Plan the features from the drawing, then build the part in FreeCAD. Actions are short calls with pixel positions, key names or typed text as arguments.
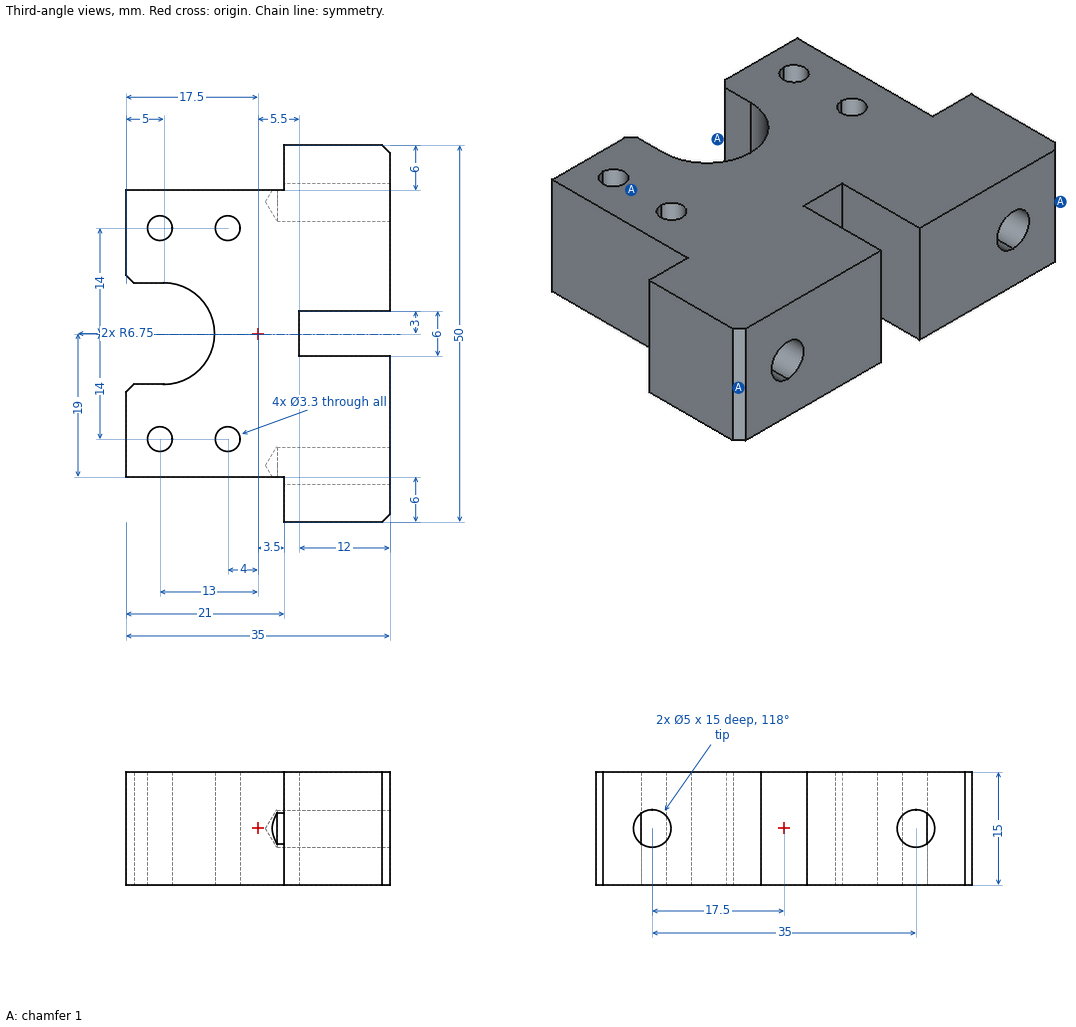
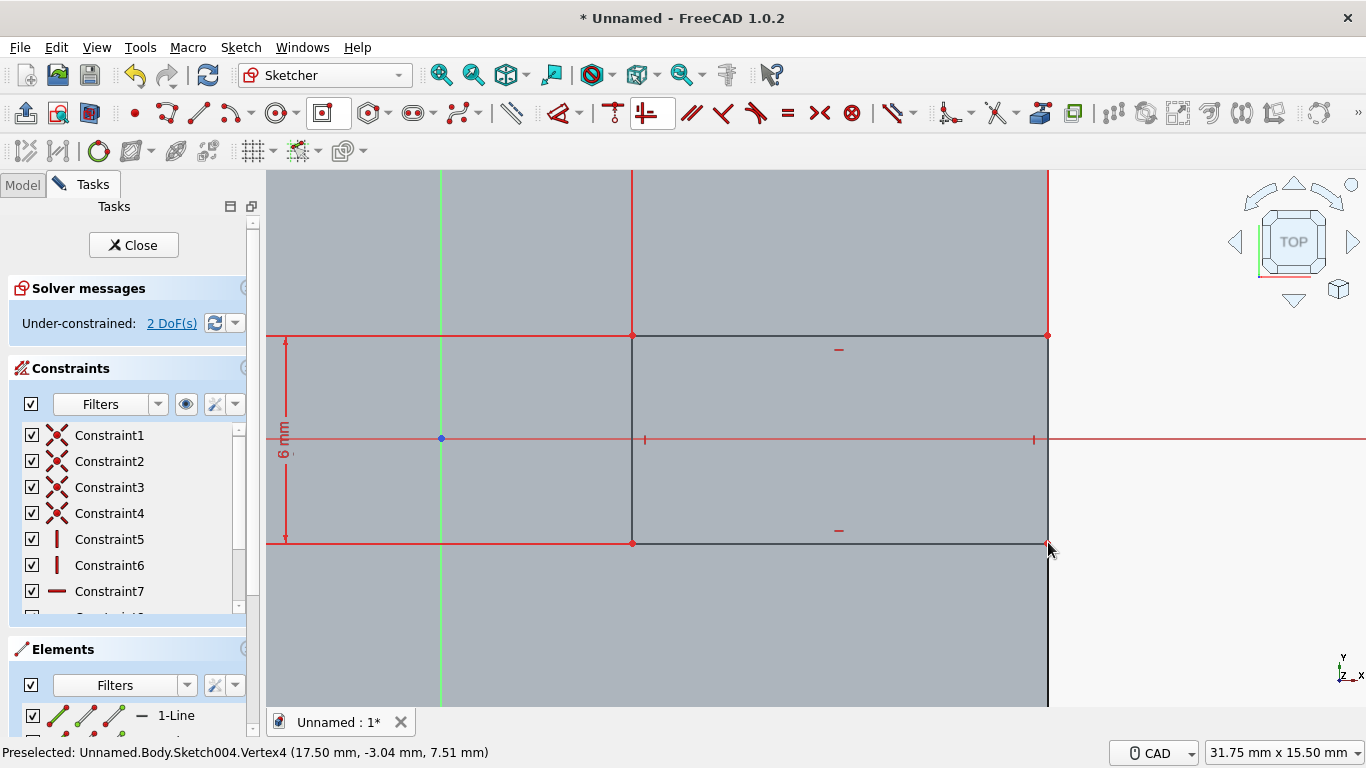
click(558, 114)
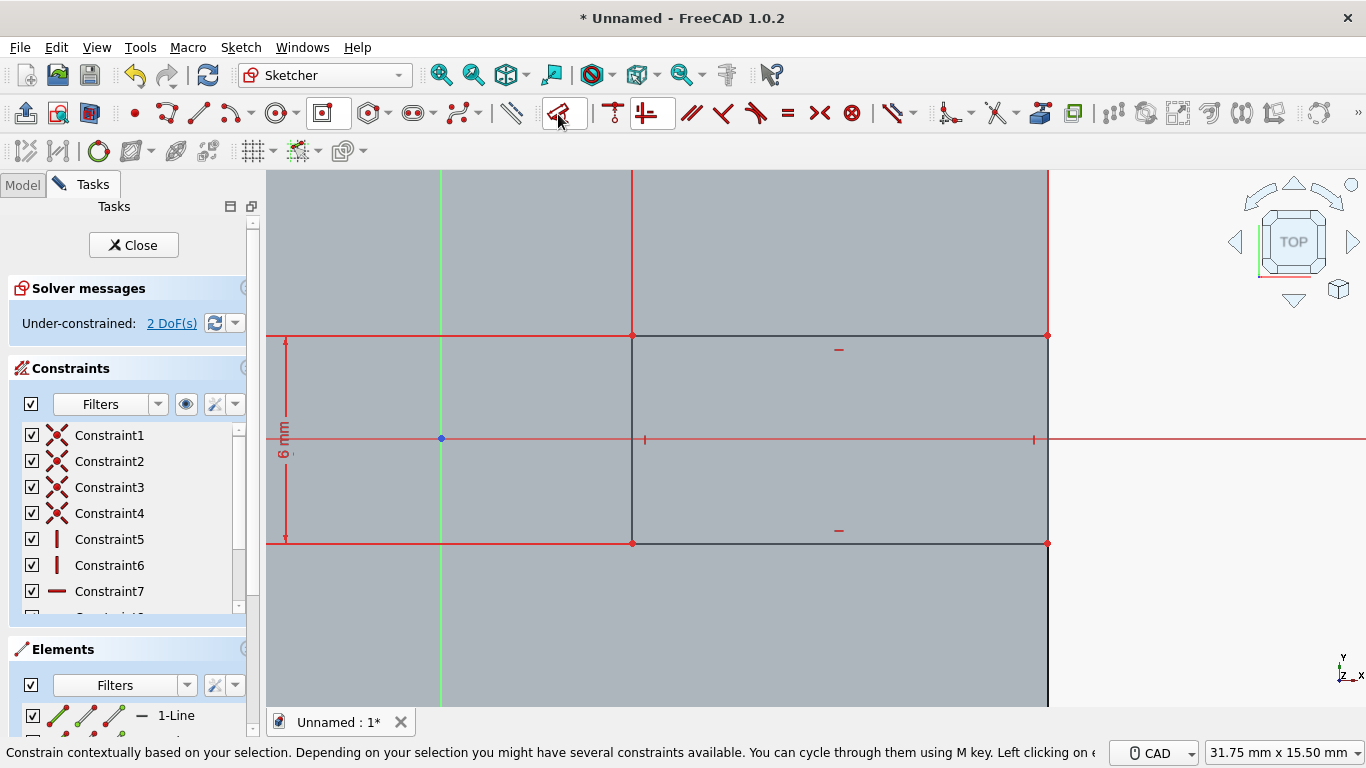
click(632, 336)
click(407, 387)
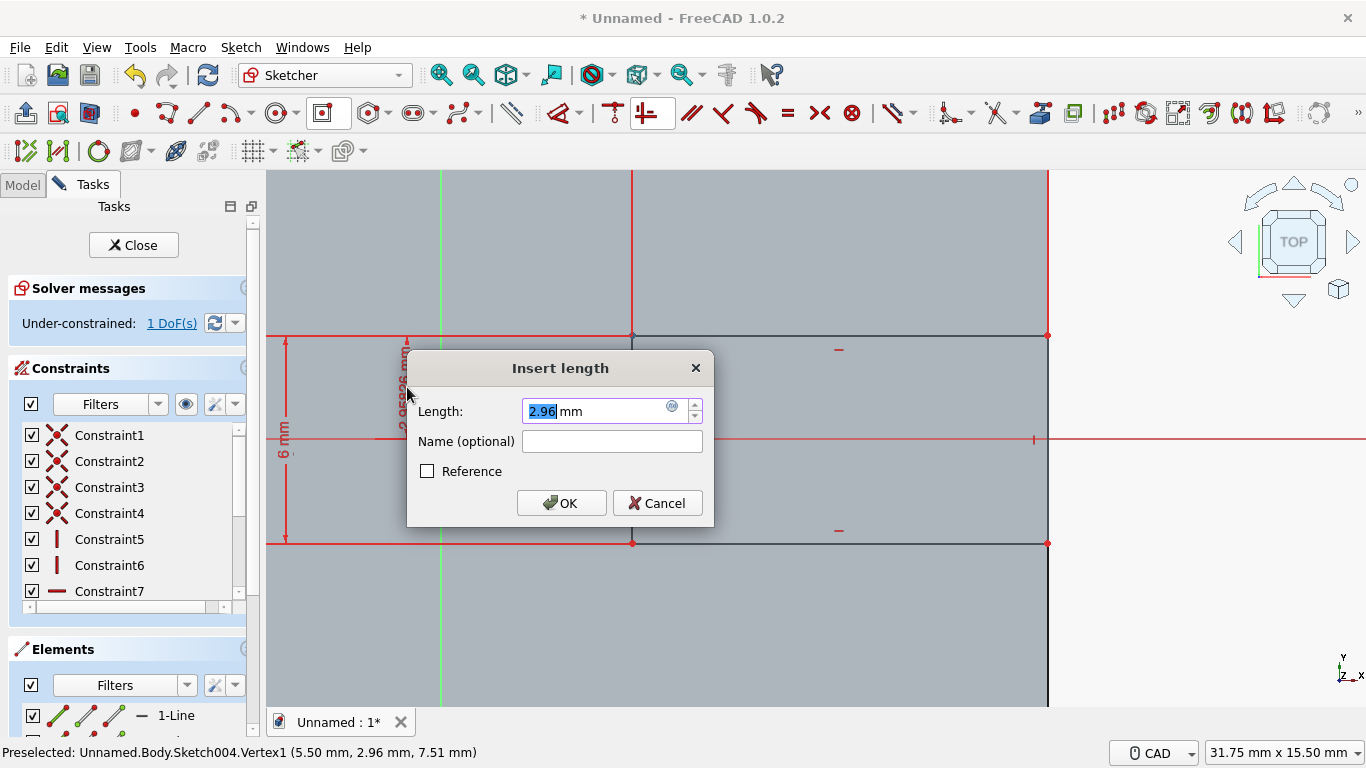
text(3)
key(Return)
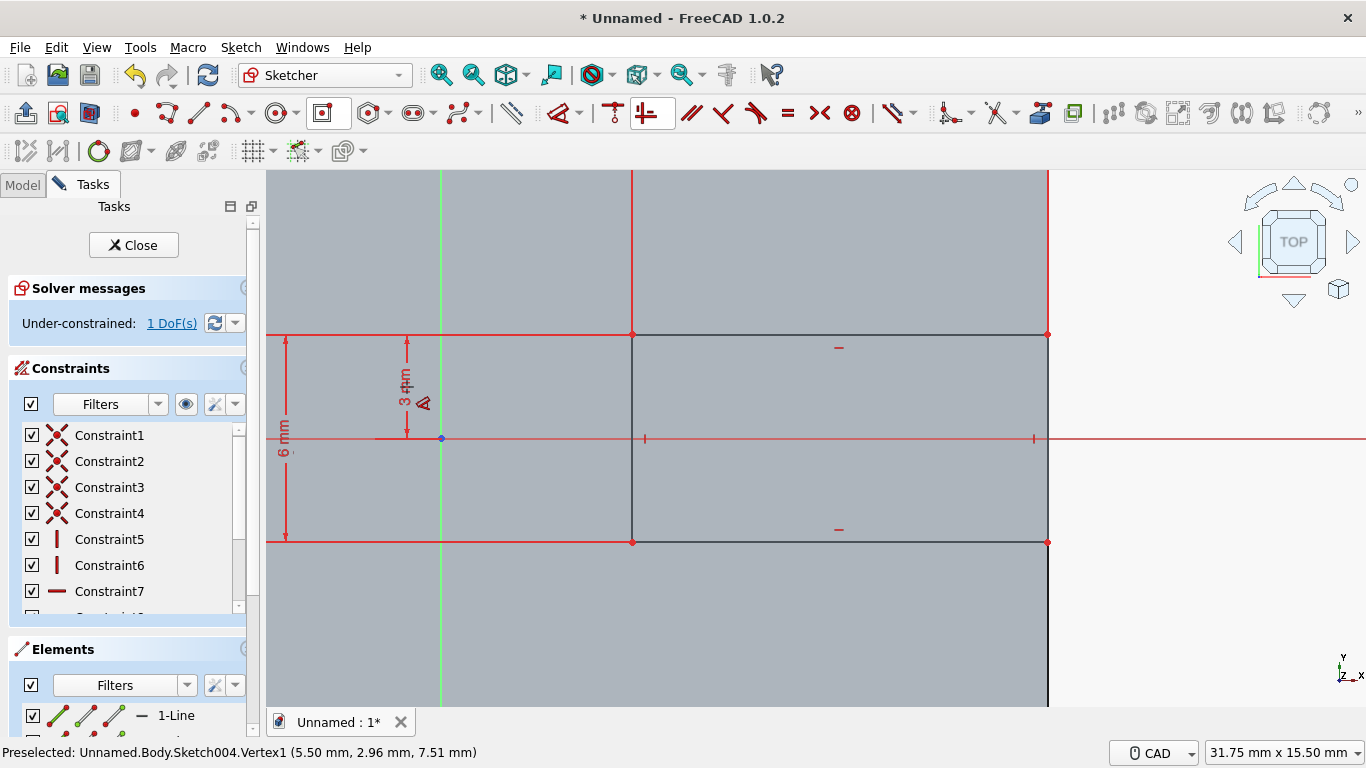
click(632, 335)
click(537, 301)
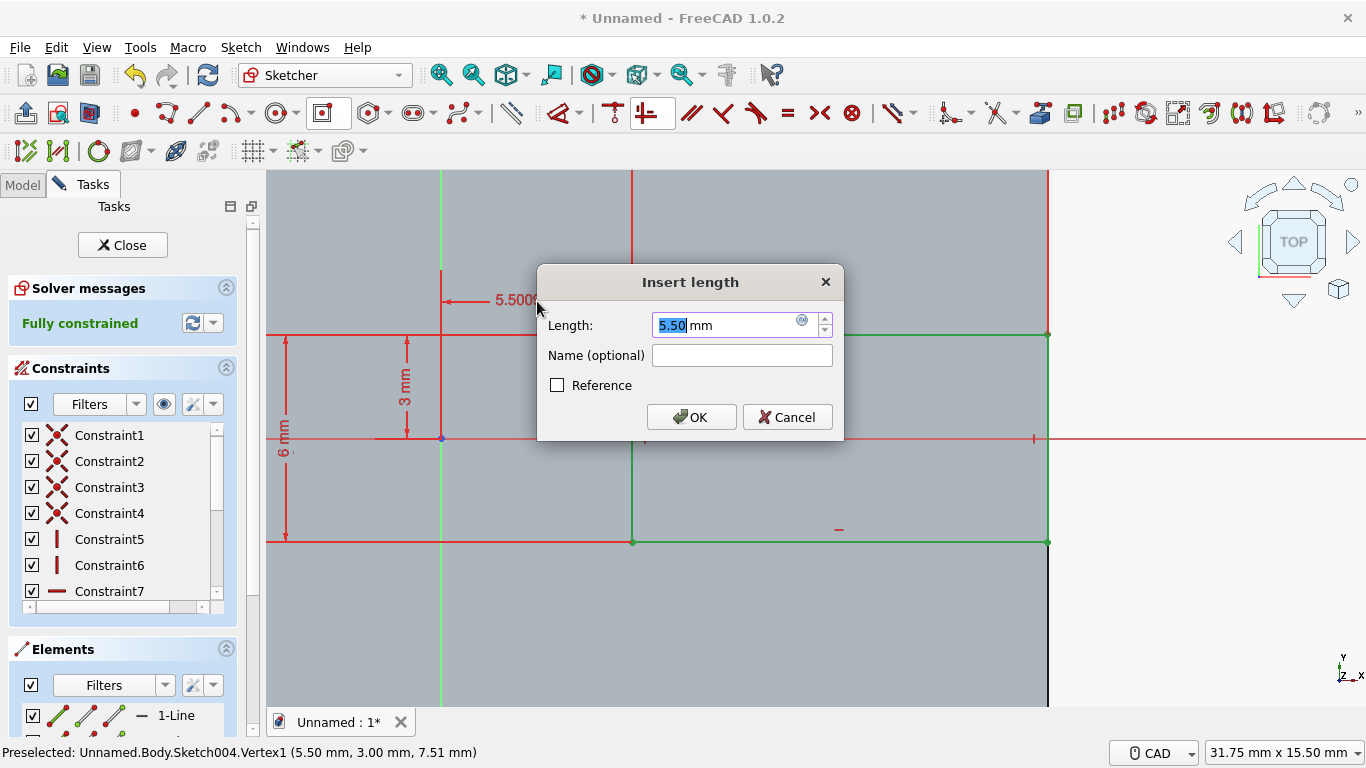
text(5.5)
key(Return)
key(Escape)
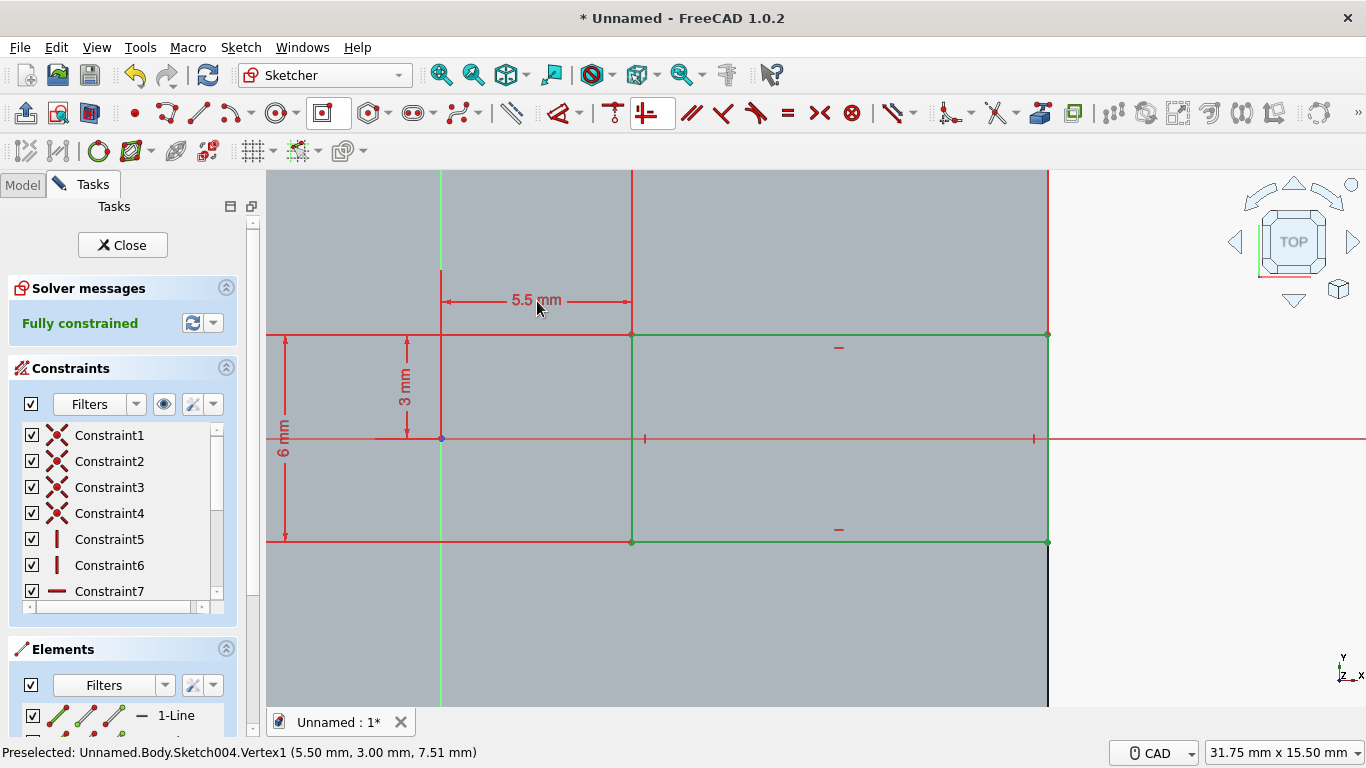
click(123, 245)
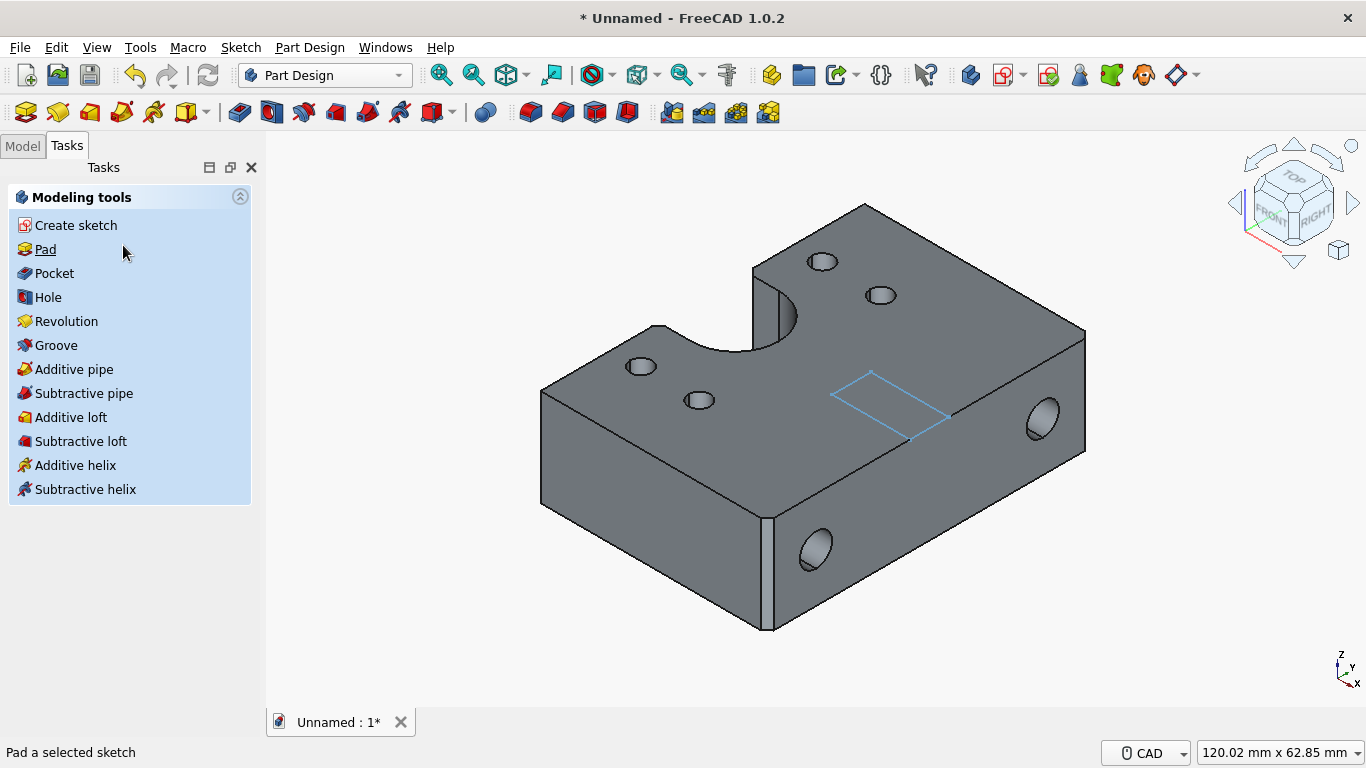
click(240, 112)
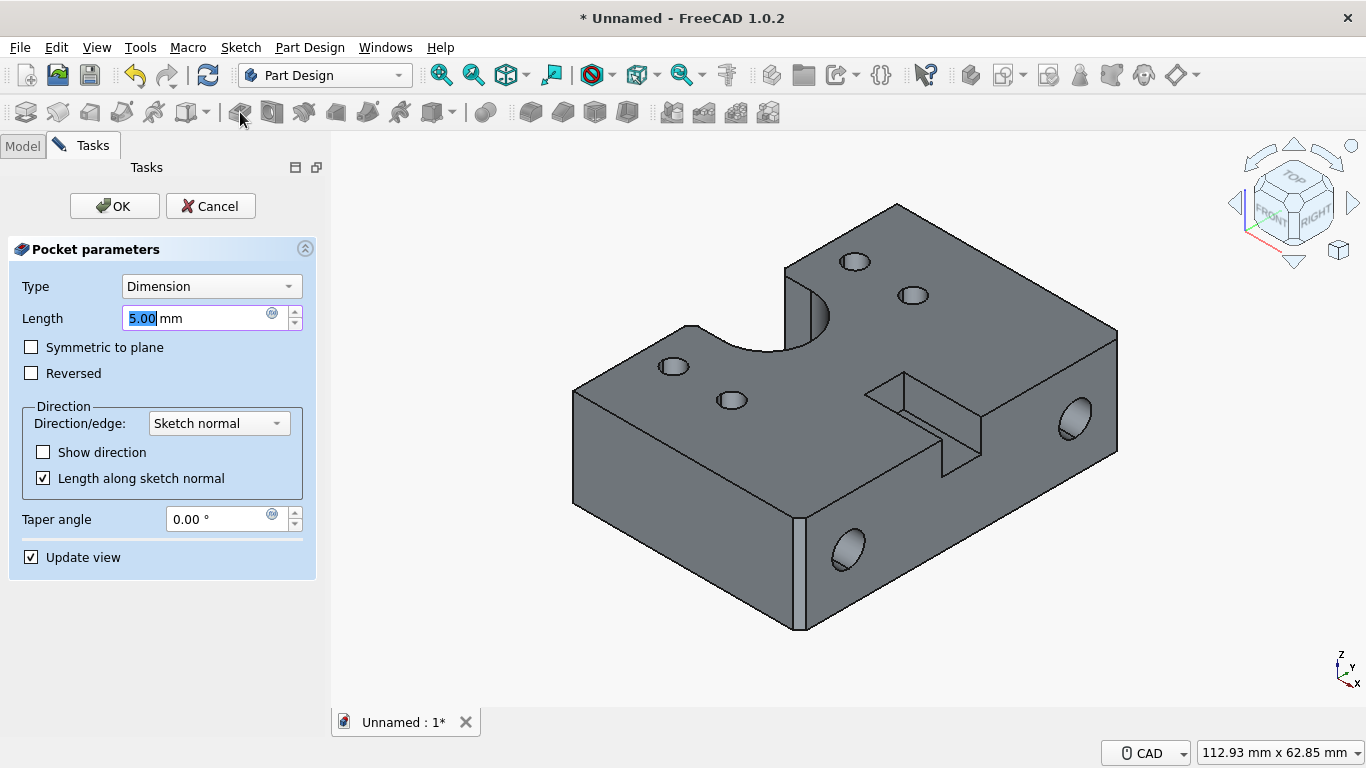
click(212, 286)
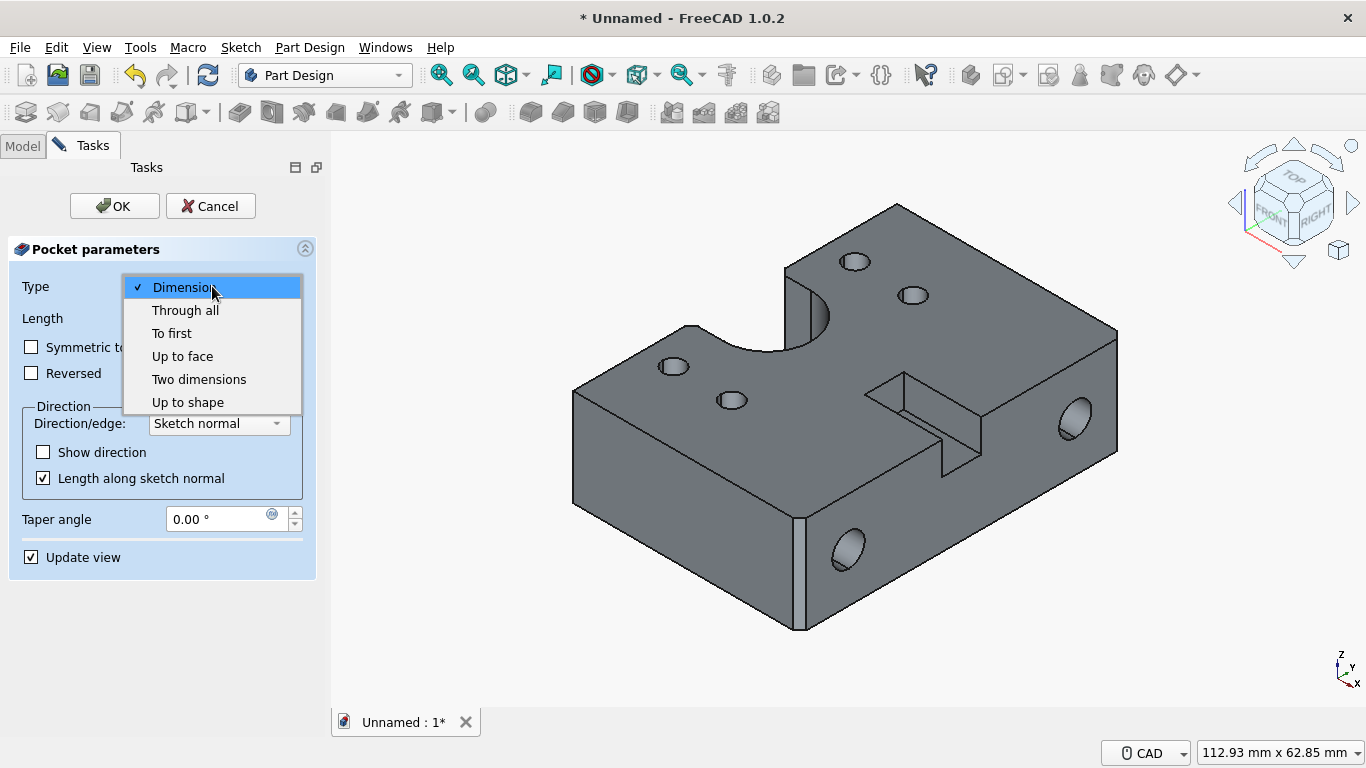
click(212, 310)